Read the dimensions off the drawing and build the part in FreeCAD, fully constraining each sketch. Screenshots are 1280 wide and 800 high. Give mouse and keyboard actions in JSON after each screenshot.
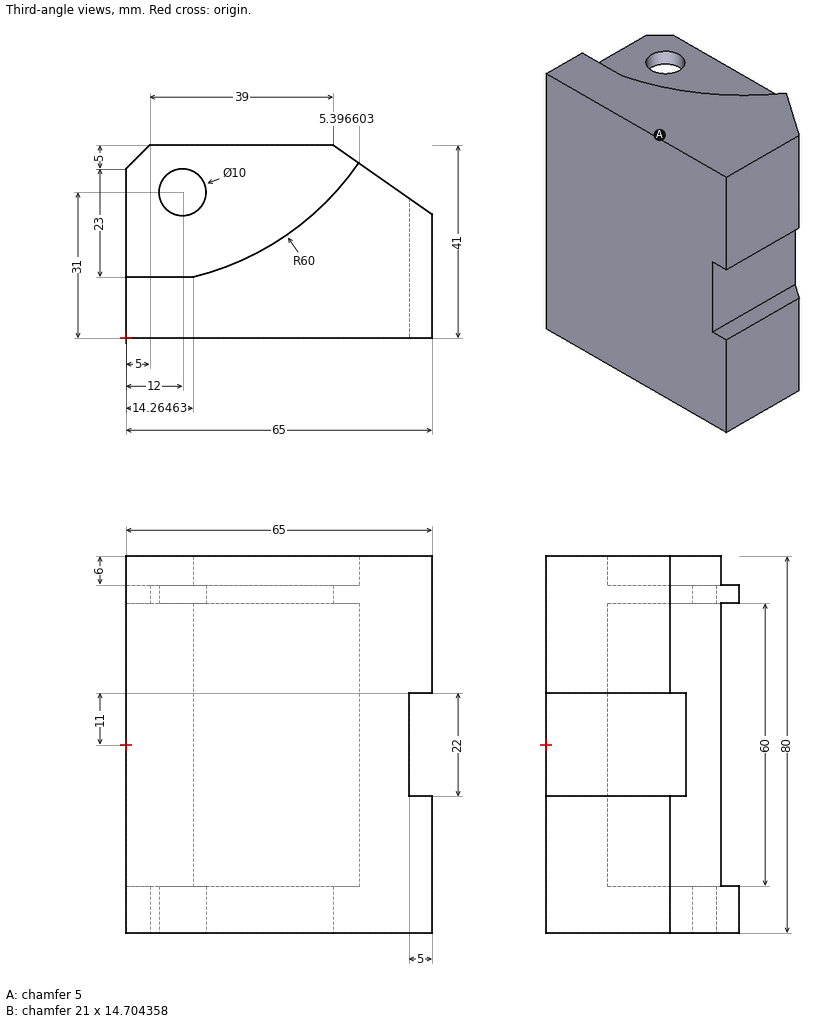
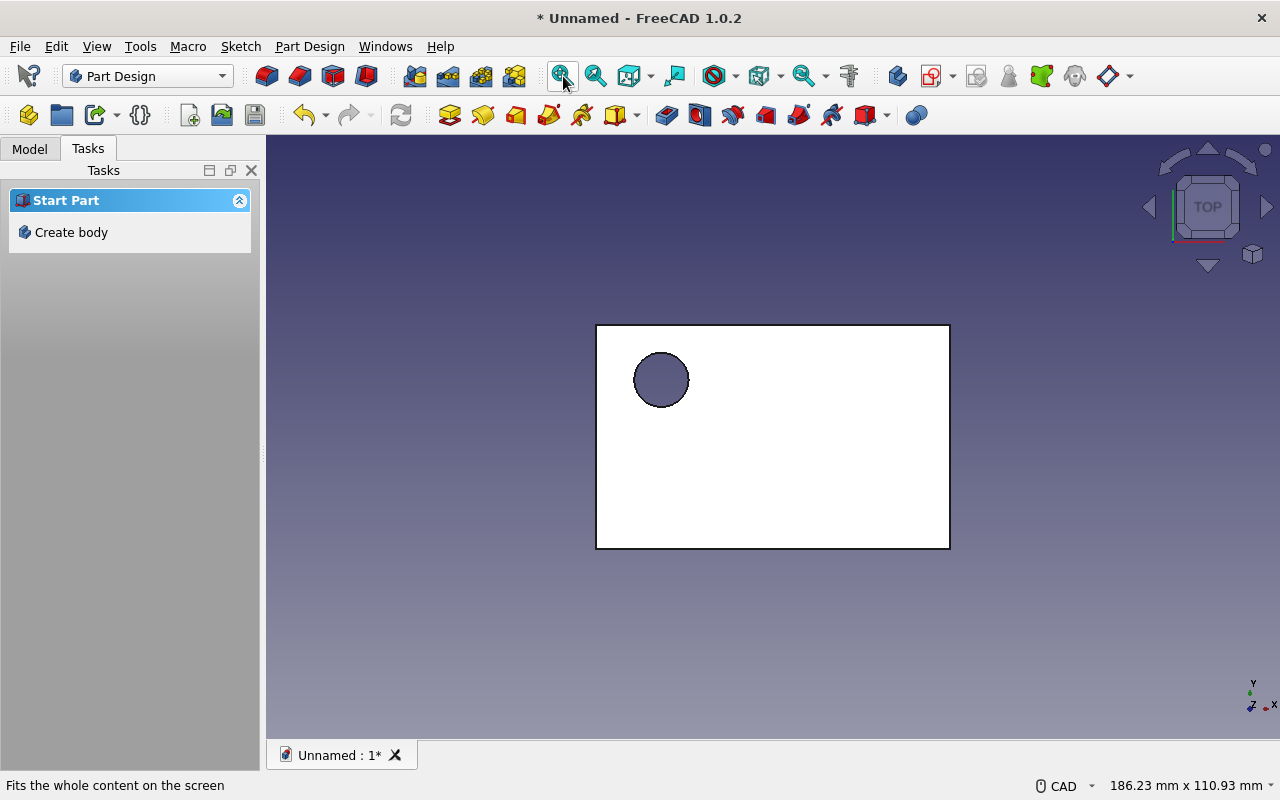
{"action": "key", "text": "1"}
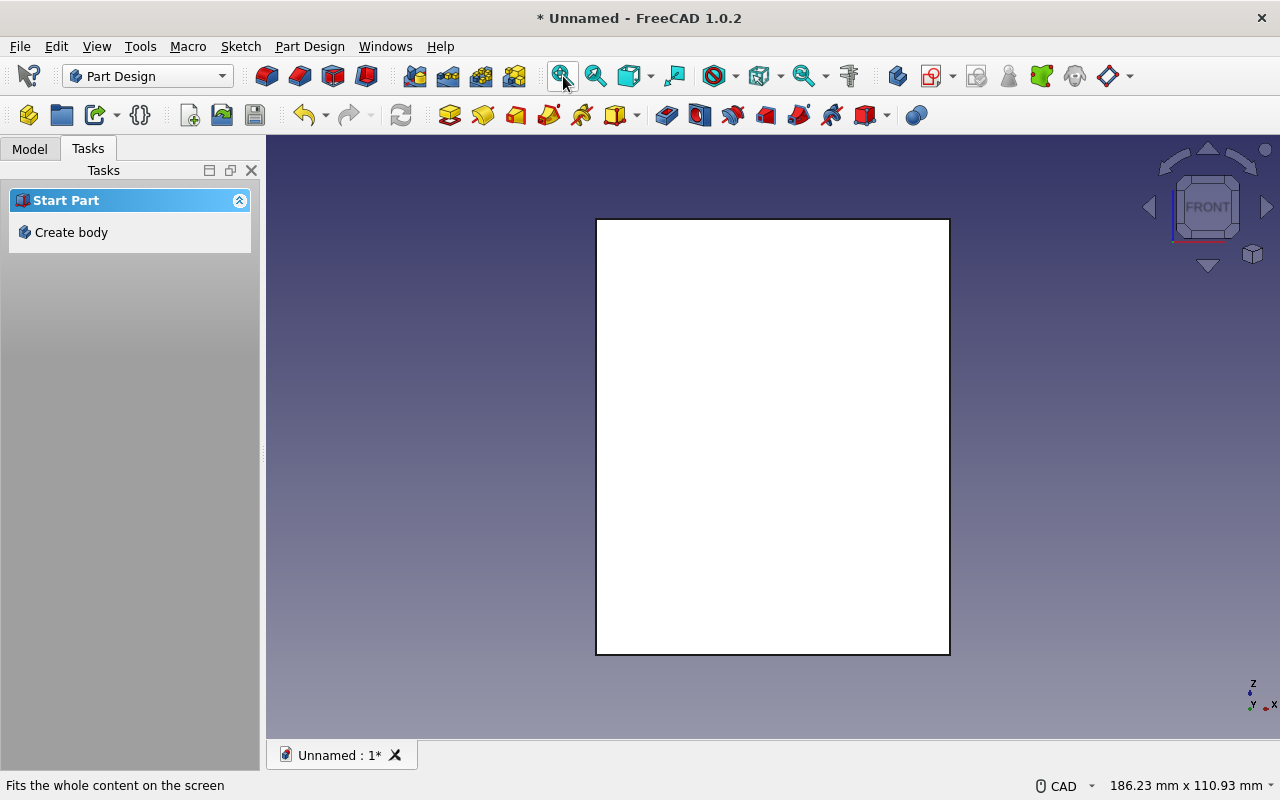
{"action": "key", "text": "3"}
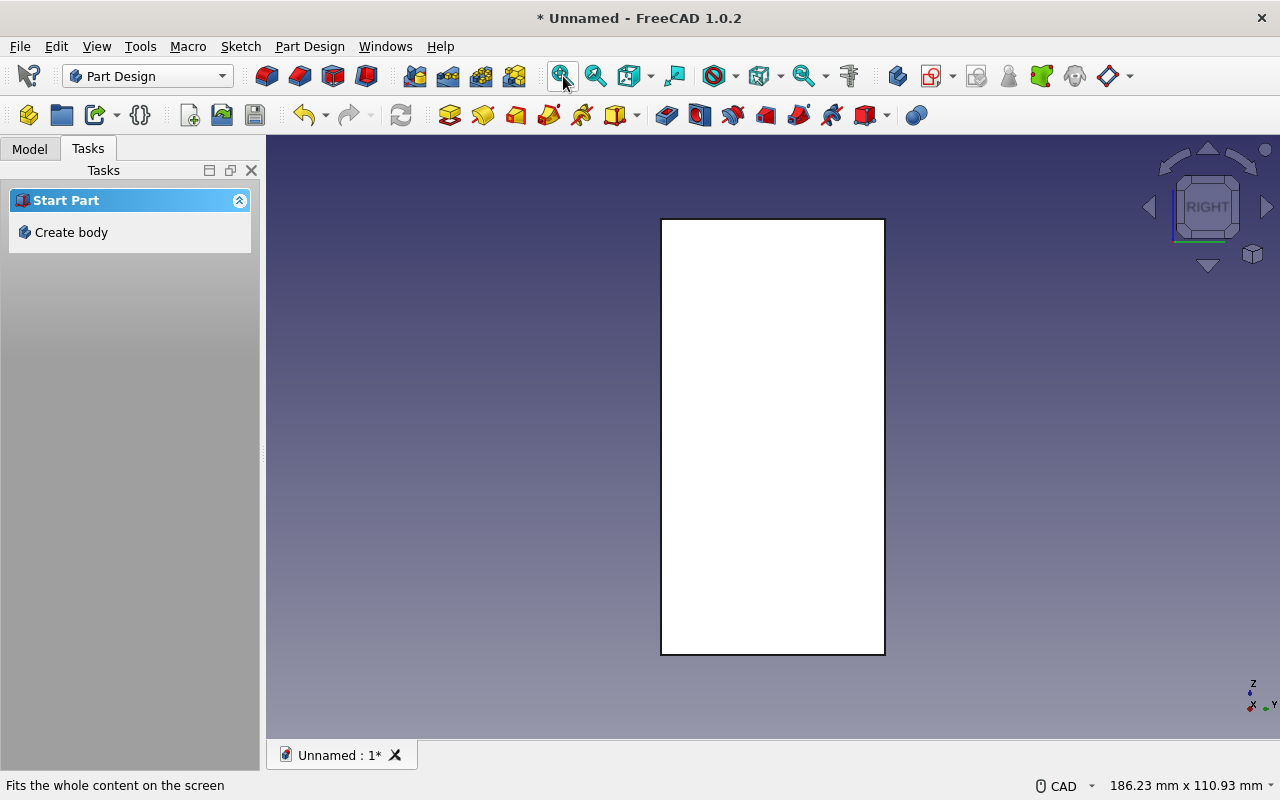
{"action": "key", "text": "5"}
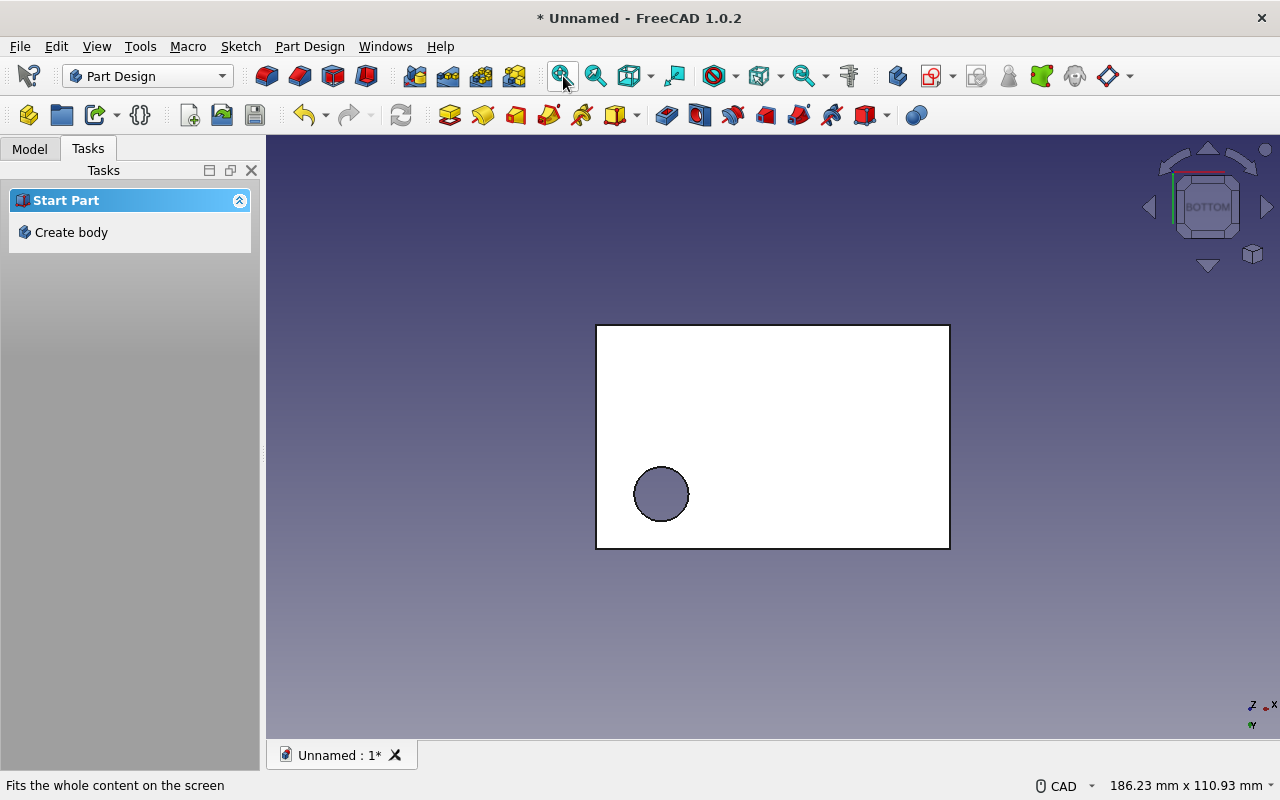
{"action": "key", "text": "v f"}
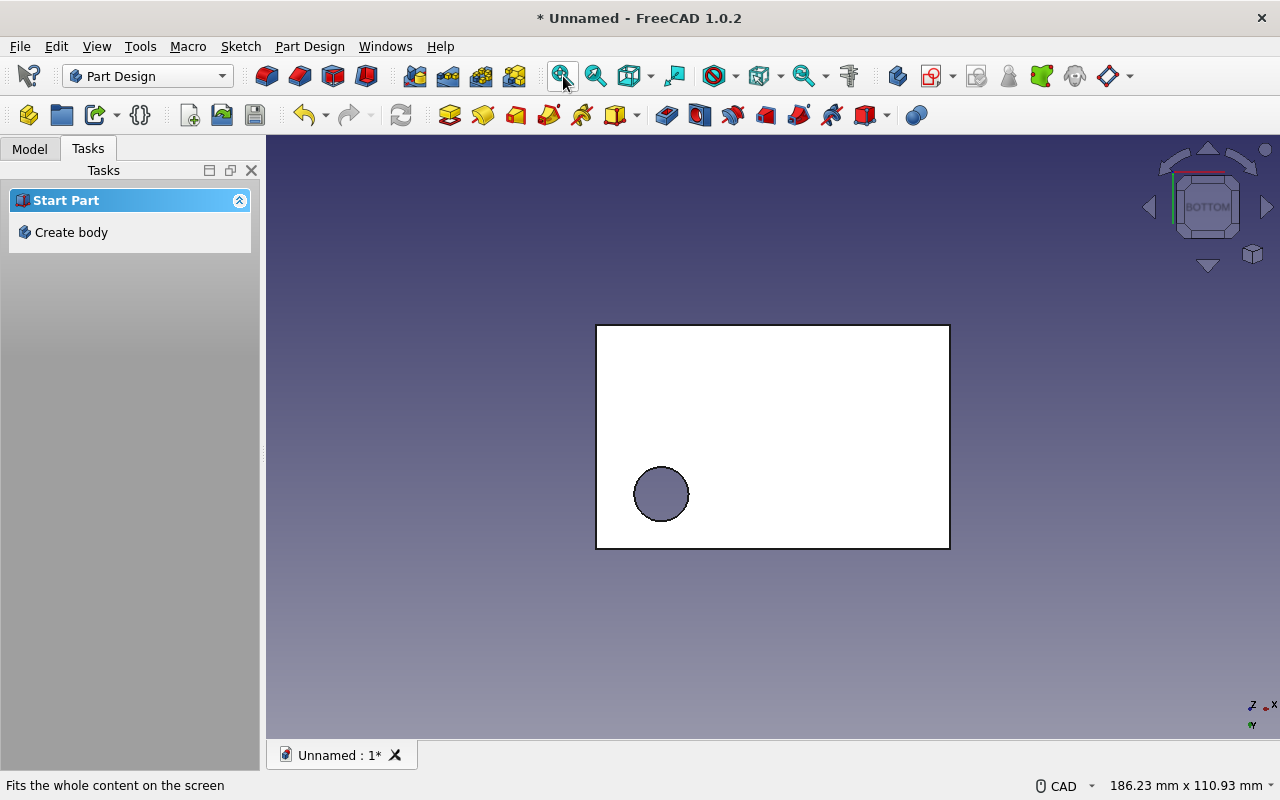
{"action": "key", "text": "4"}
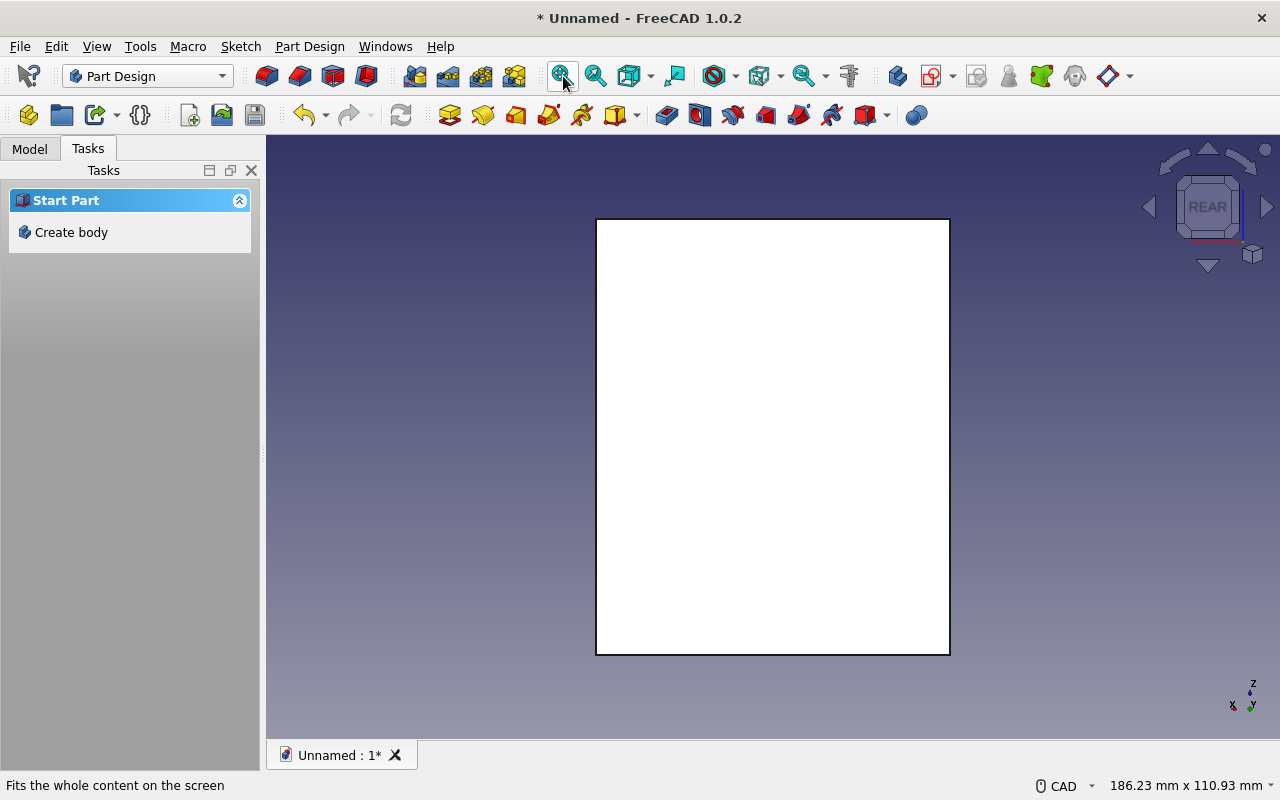
{"action": "left_click", "coordinate": [950, 436]}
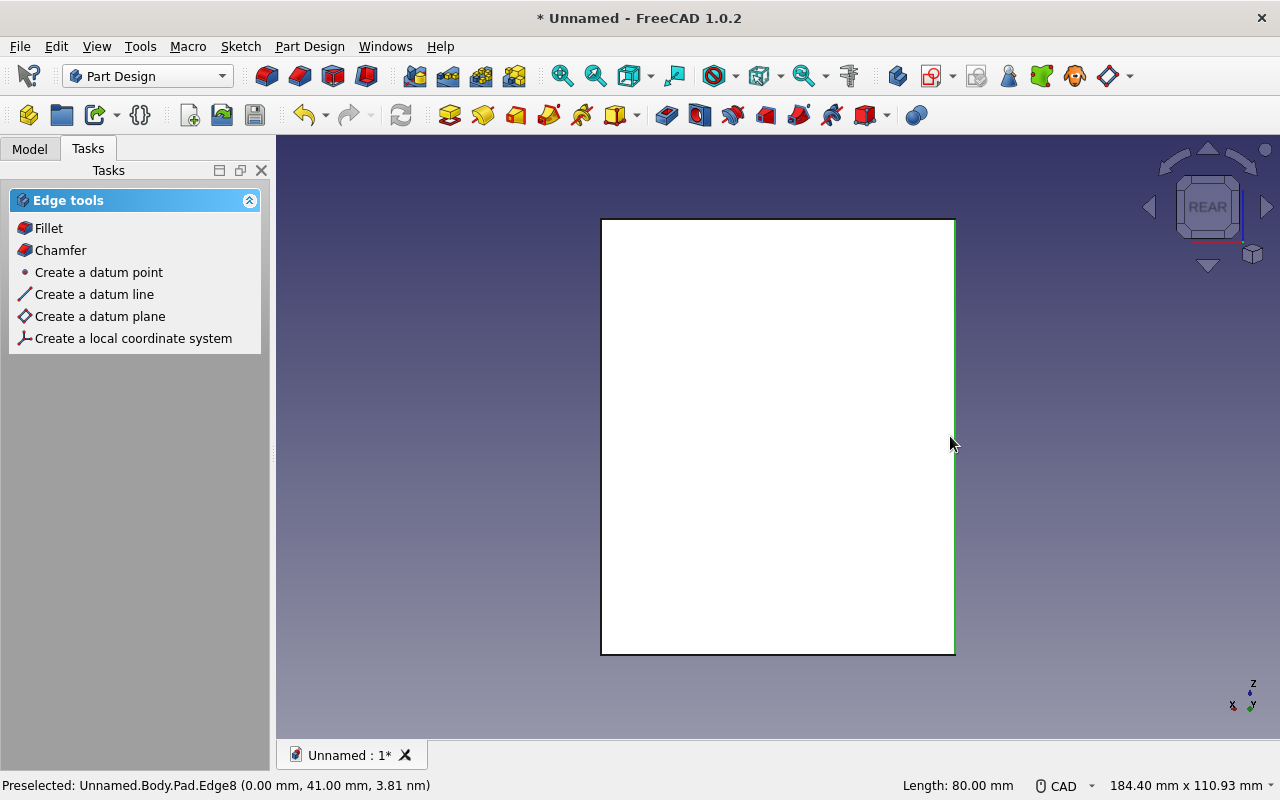
{"action": "left_click", "coordinate": [300, 76]}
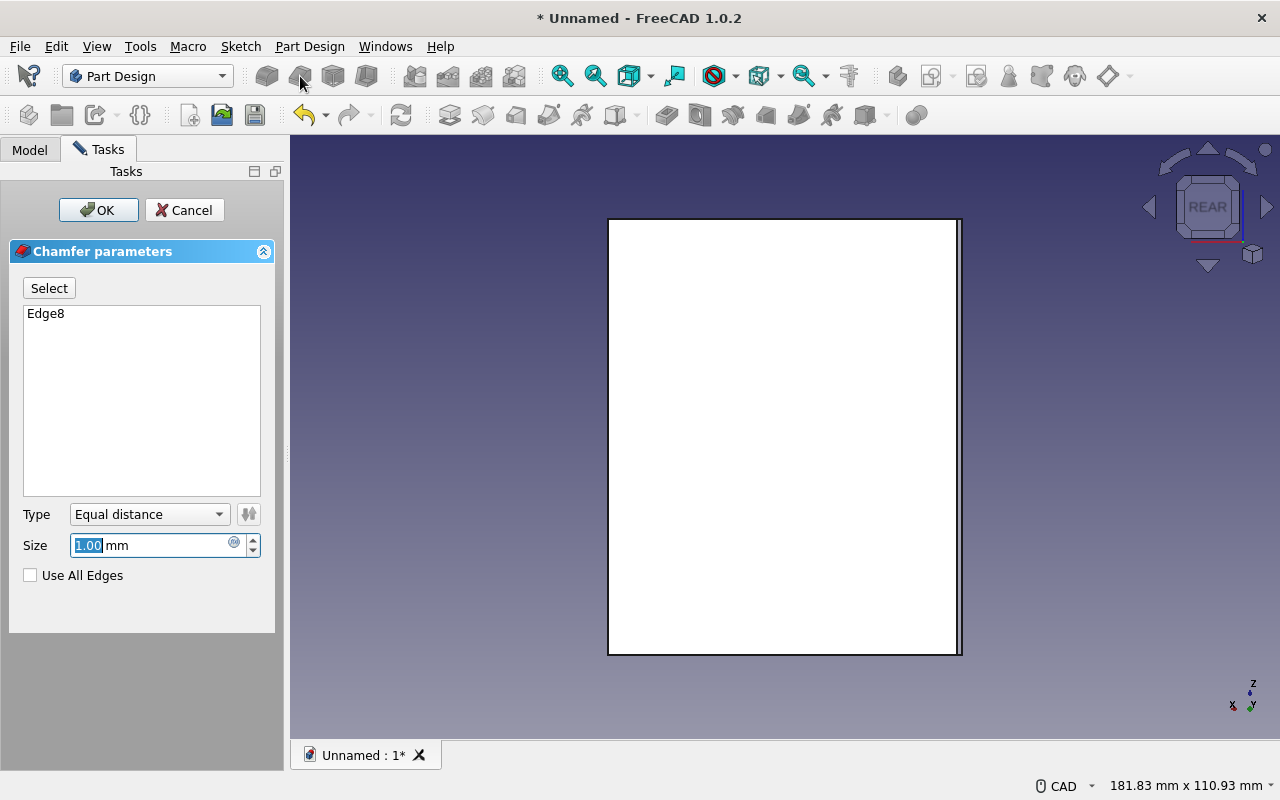
{"action": "type", "text": "5"}
{"action": "key", "text": "Tab"}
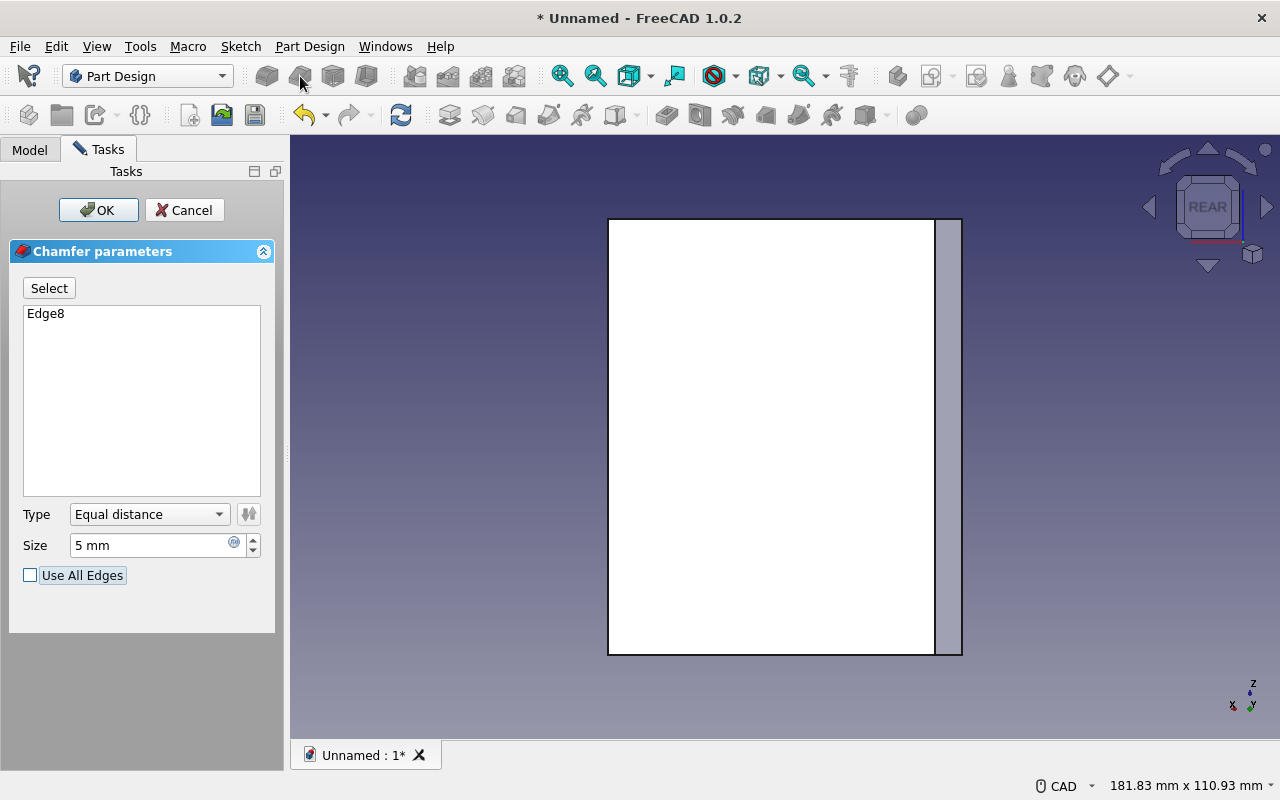
{"action": "left_click", "coordinate": [99, 210]}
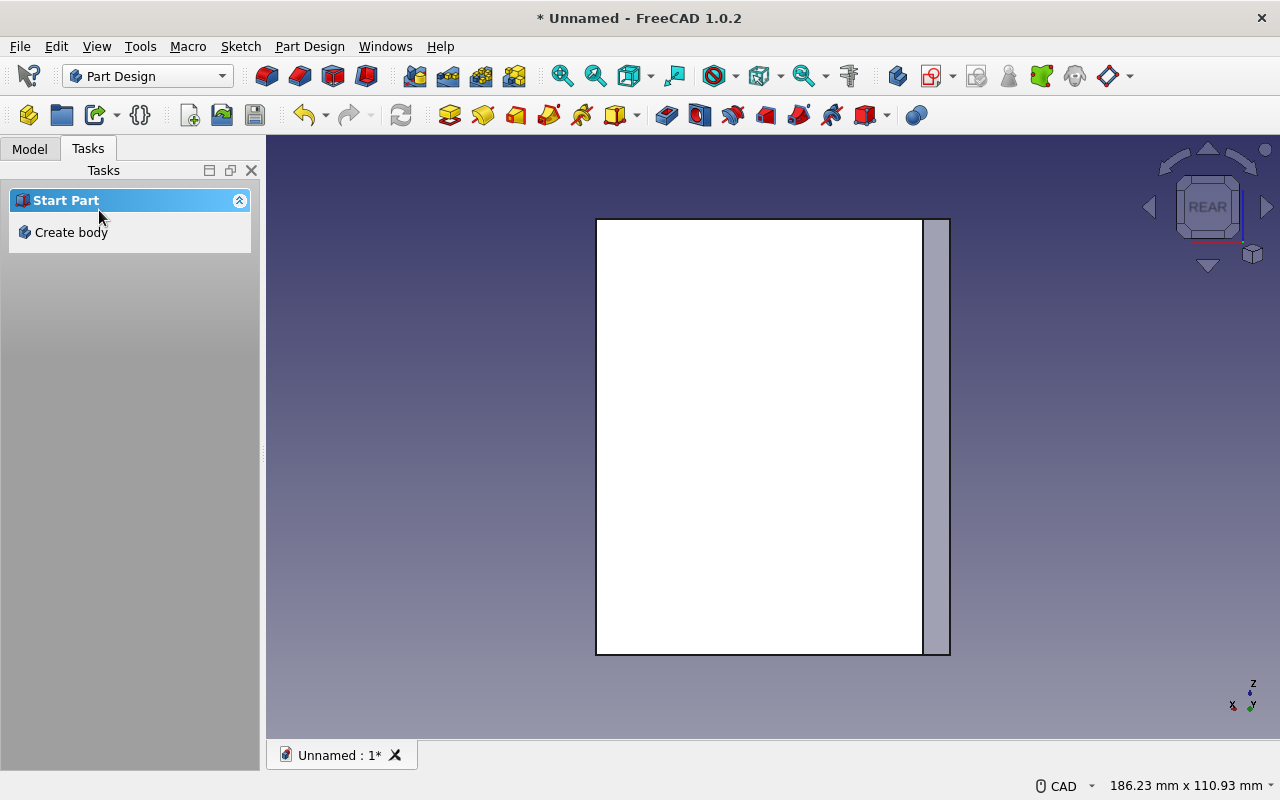
{"action": "left_click", "coordinate": [596, 436]}